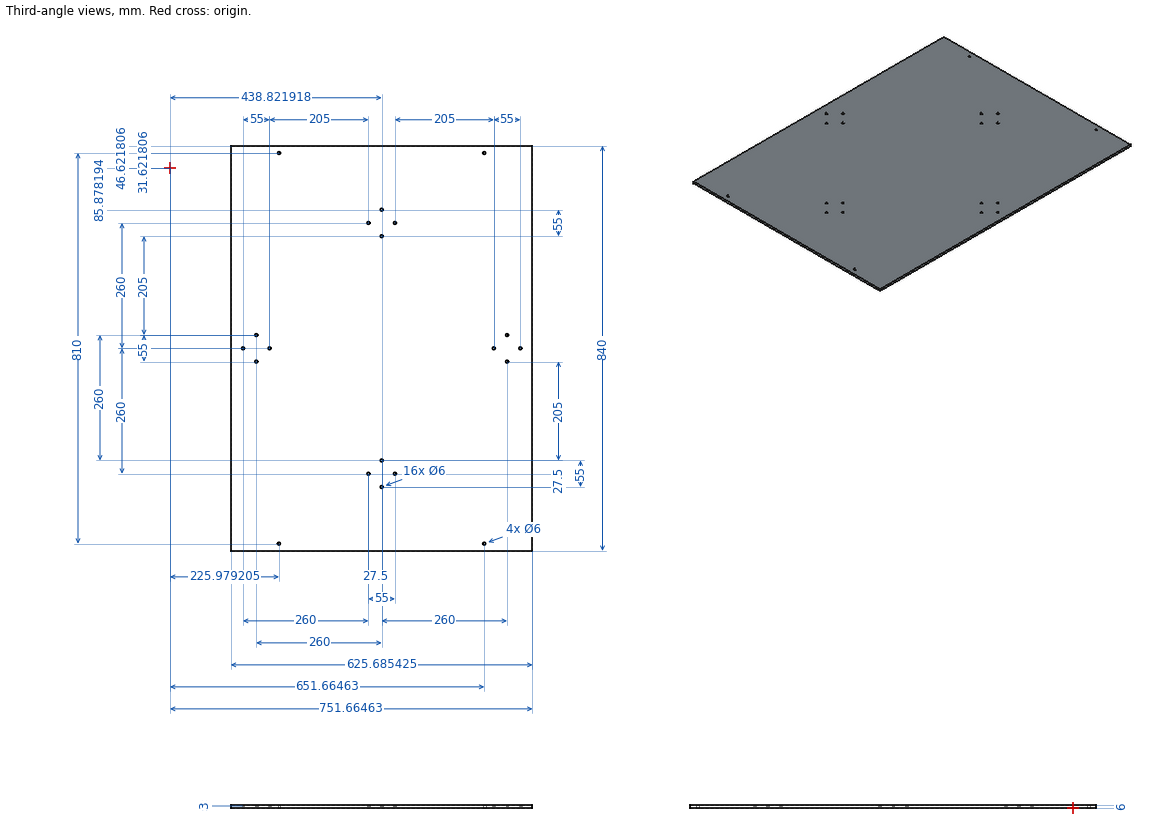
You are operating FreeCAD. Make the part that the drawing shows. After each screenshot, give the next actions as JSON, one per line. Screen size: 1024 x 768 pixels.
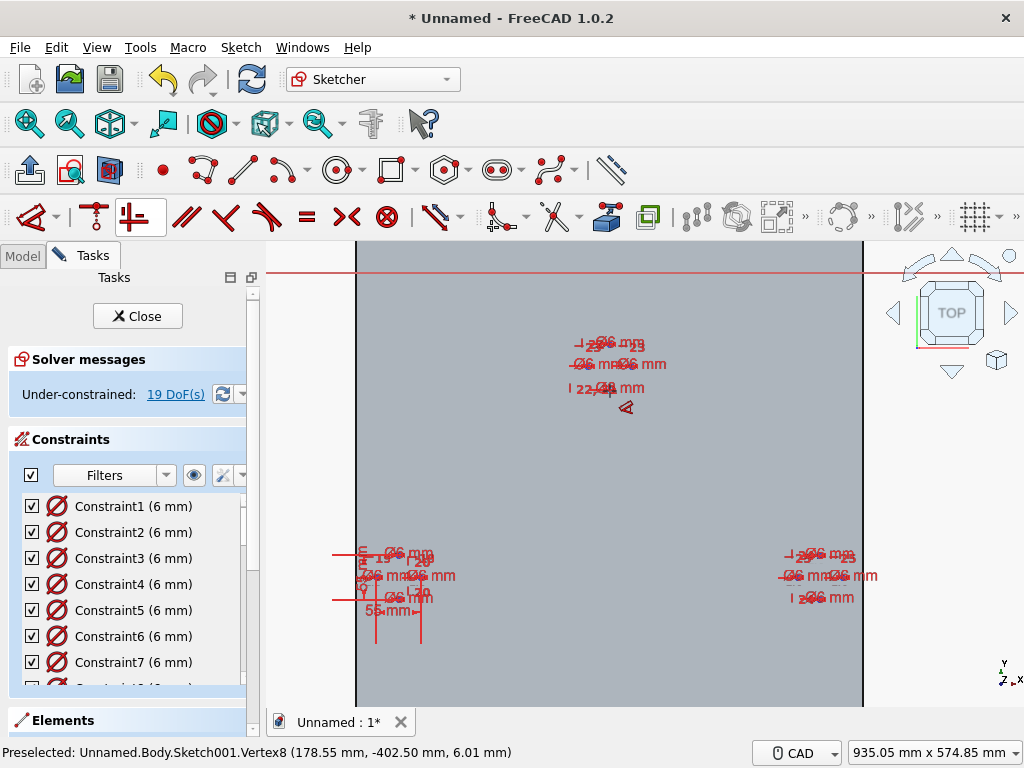
{"action": "left_click", "coordinate": [610, 390]}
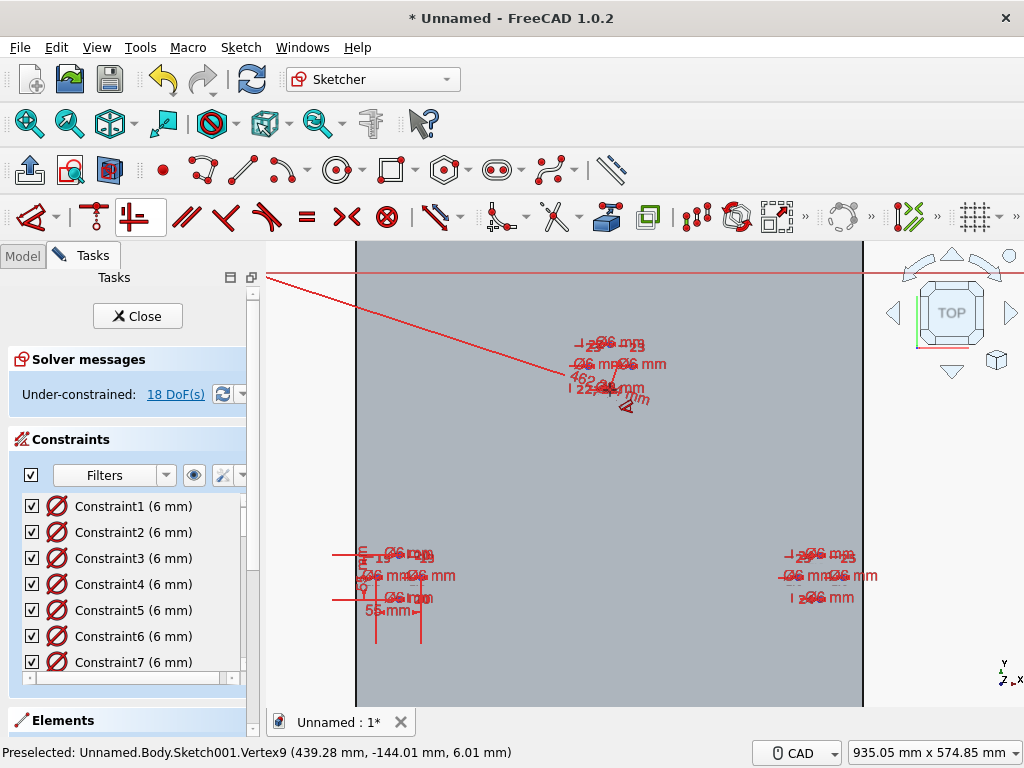
{"action": "left_click", "coordinate": [610, 344]}
{"action": "left_click", "coordinate": [644, 357]}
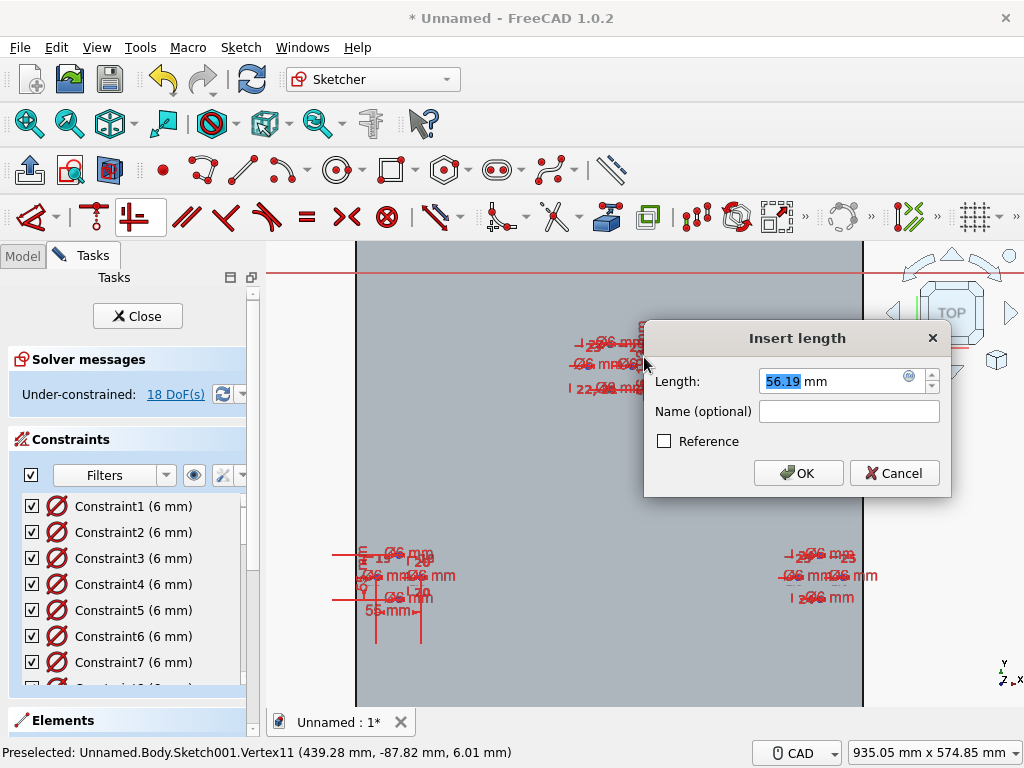
{"action": "type", "text": "55"}
{"action": "key", "text": "Return"}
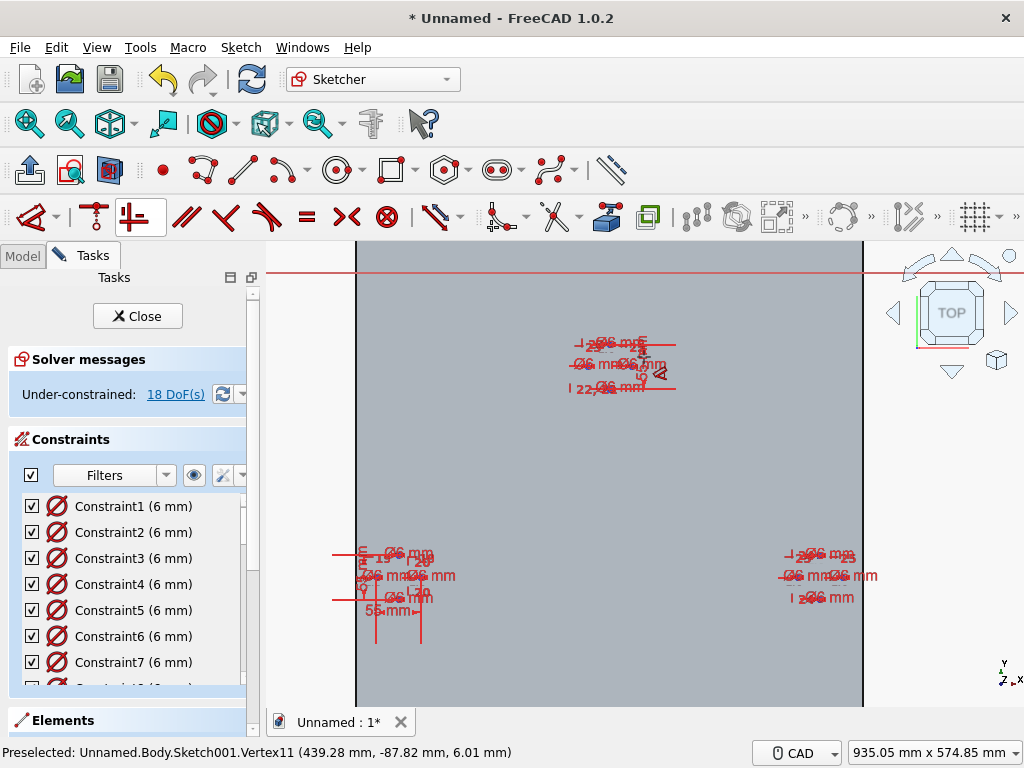
{"action": "left_click", "coordinate": [588, 366]}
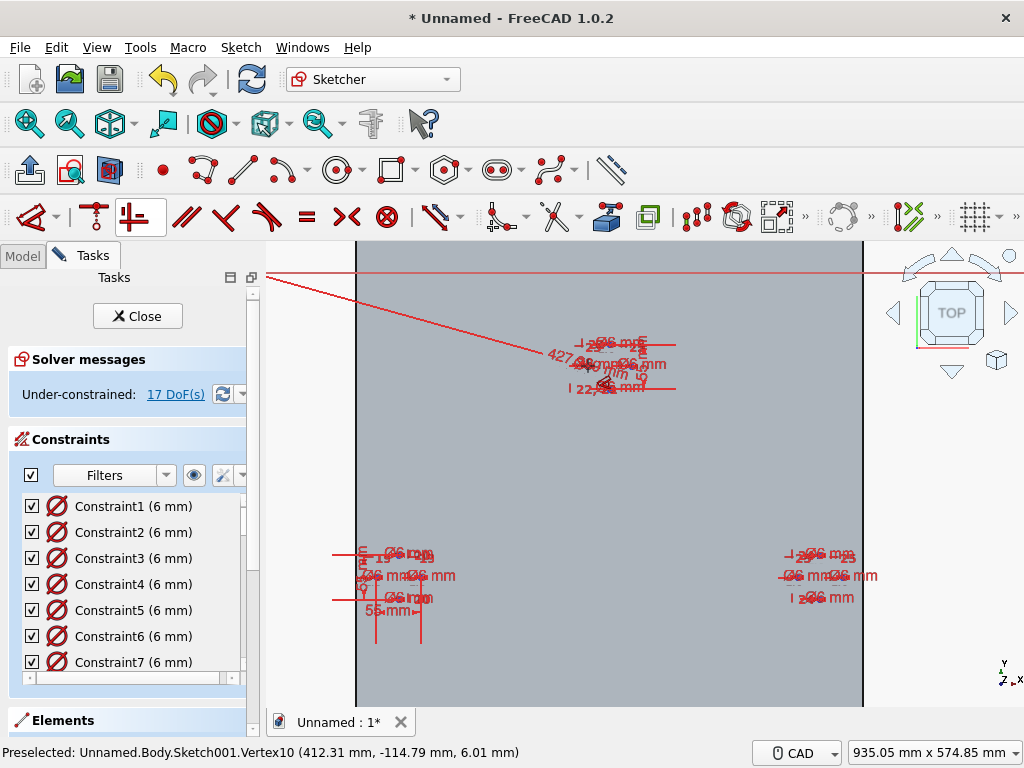
{"action": "left_click", "coordinate": [631, 366]}
{"action": "left_click", "coordinate": [600, 332]}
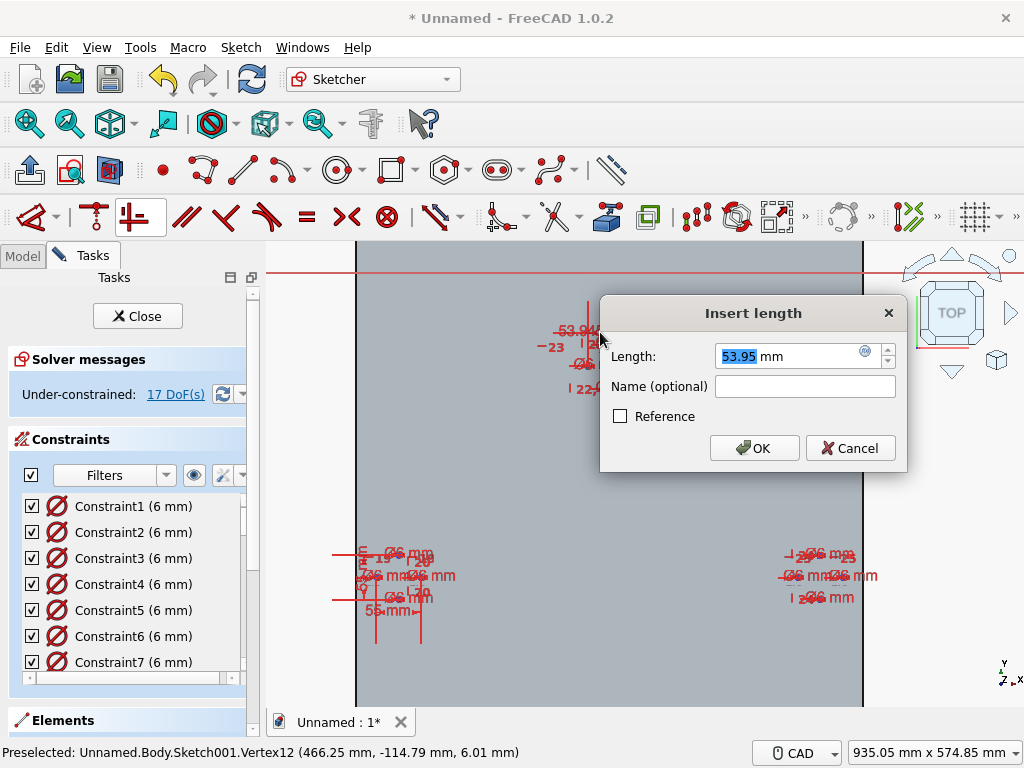
{"action": "type", "text": "55"}
{"action": "key", "text": "Return"}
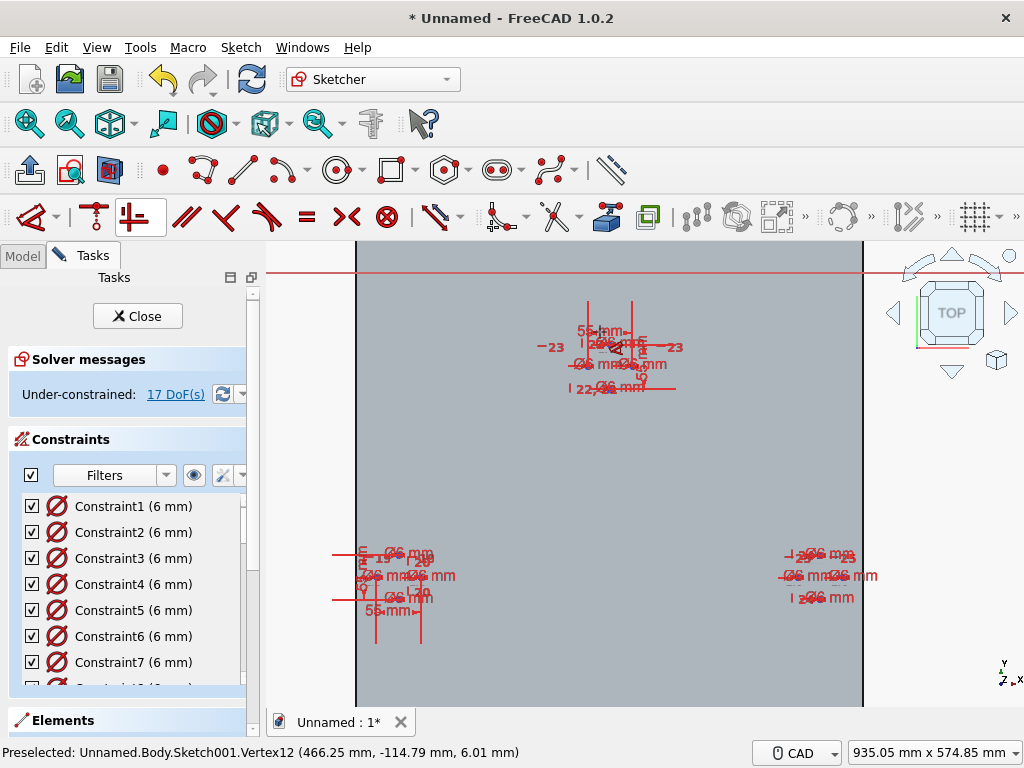
{"action": "left_click", "coordinate": [819, 599]}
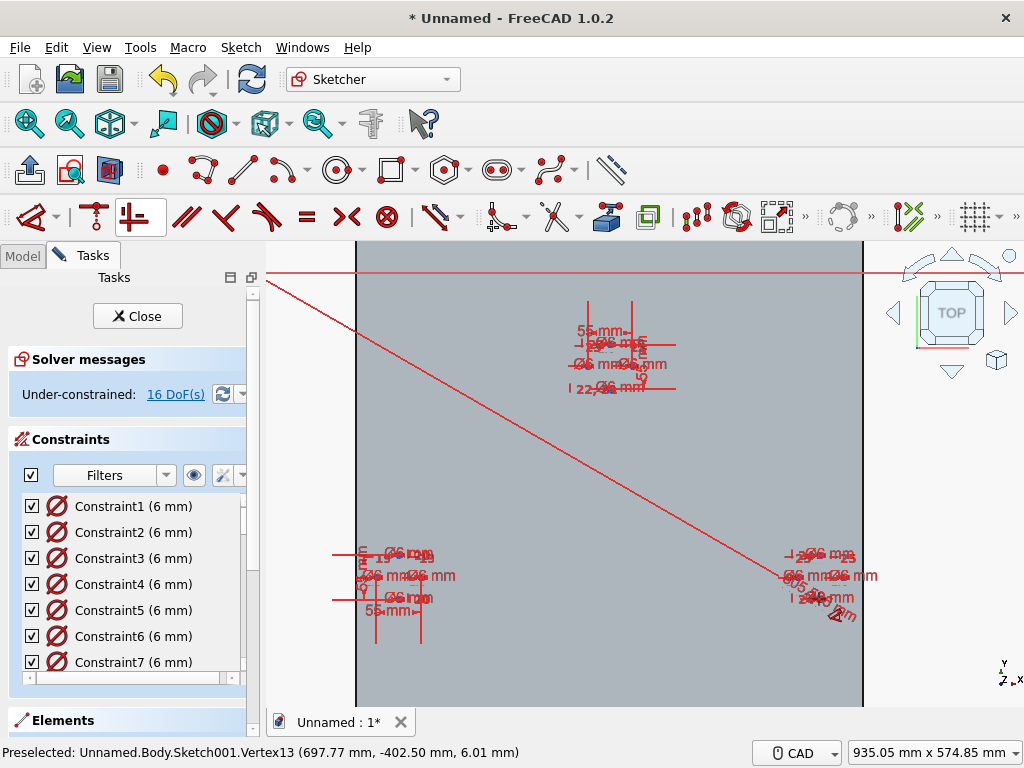
{"action": "left_click", "coordinate": [819, 556]}
{"action": "left_click", "coordinate": [853, 562]}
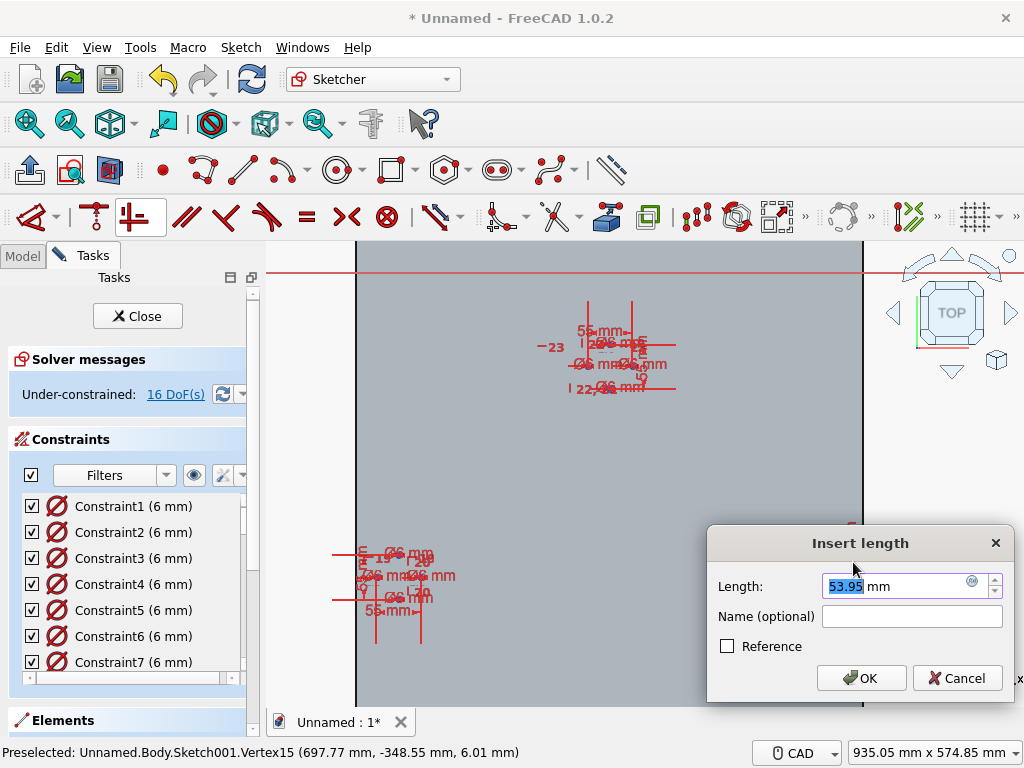
{"action": "type", "text": "55"}
{"action": "key", "text": "Return"}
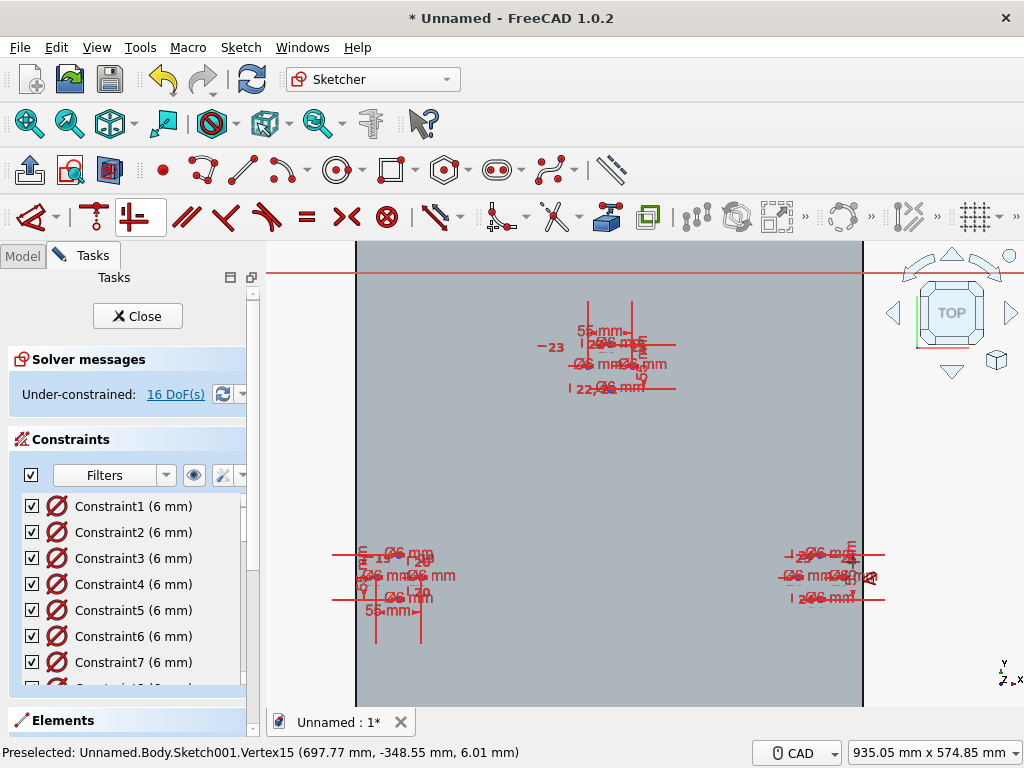
{"action": "left_click", "coordinate": [797, 578]}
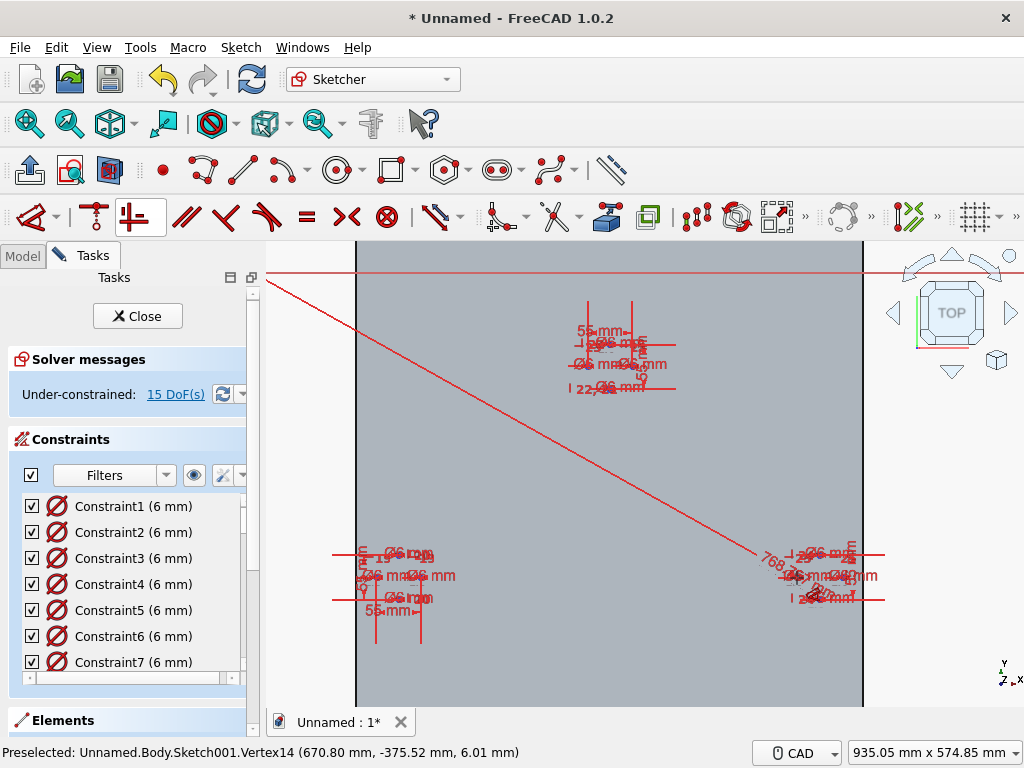
{"action": "left_click", "coordinate": [843, 578]}
{"action": "left_click", "coordinate": [831, 612]}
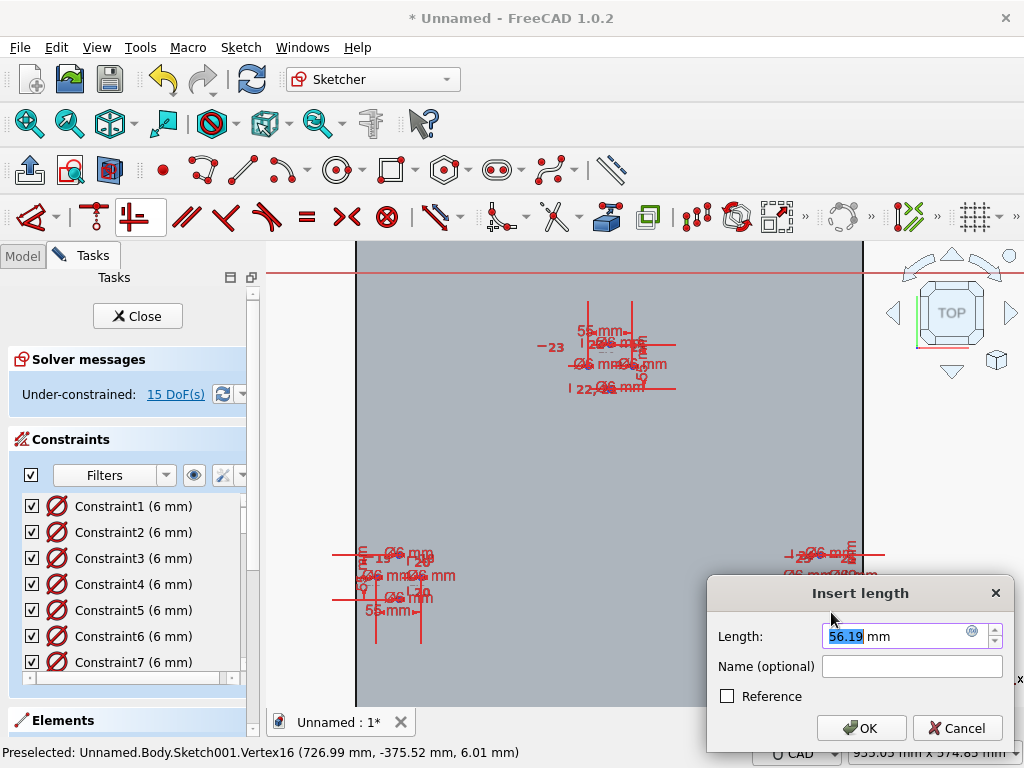
{"action": "type", "text": "55"}
{"action": "key", "text": "Return"}